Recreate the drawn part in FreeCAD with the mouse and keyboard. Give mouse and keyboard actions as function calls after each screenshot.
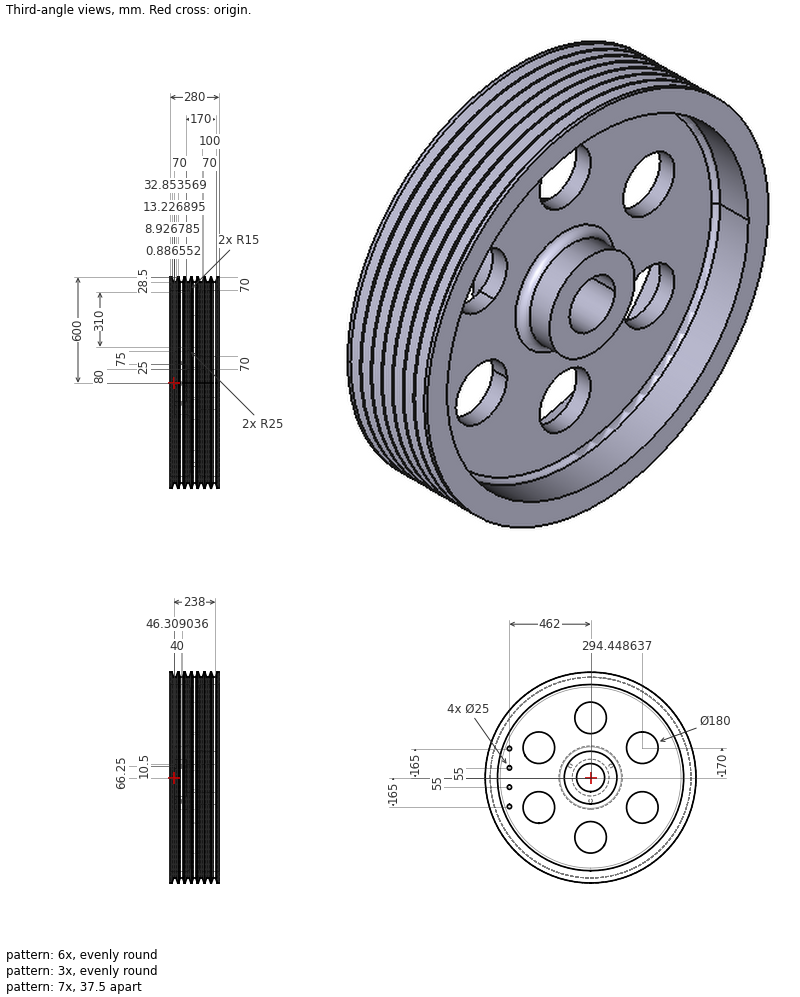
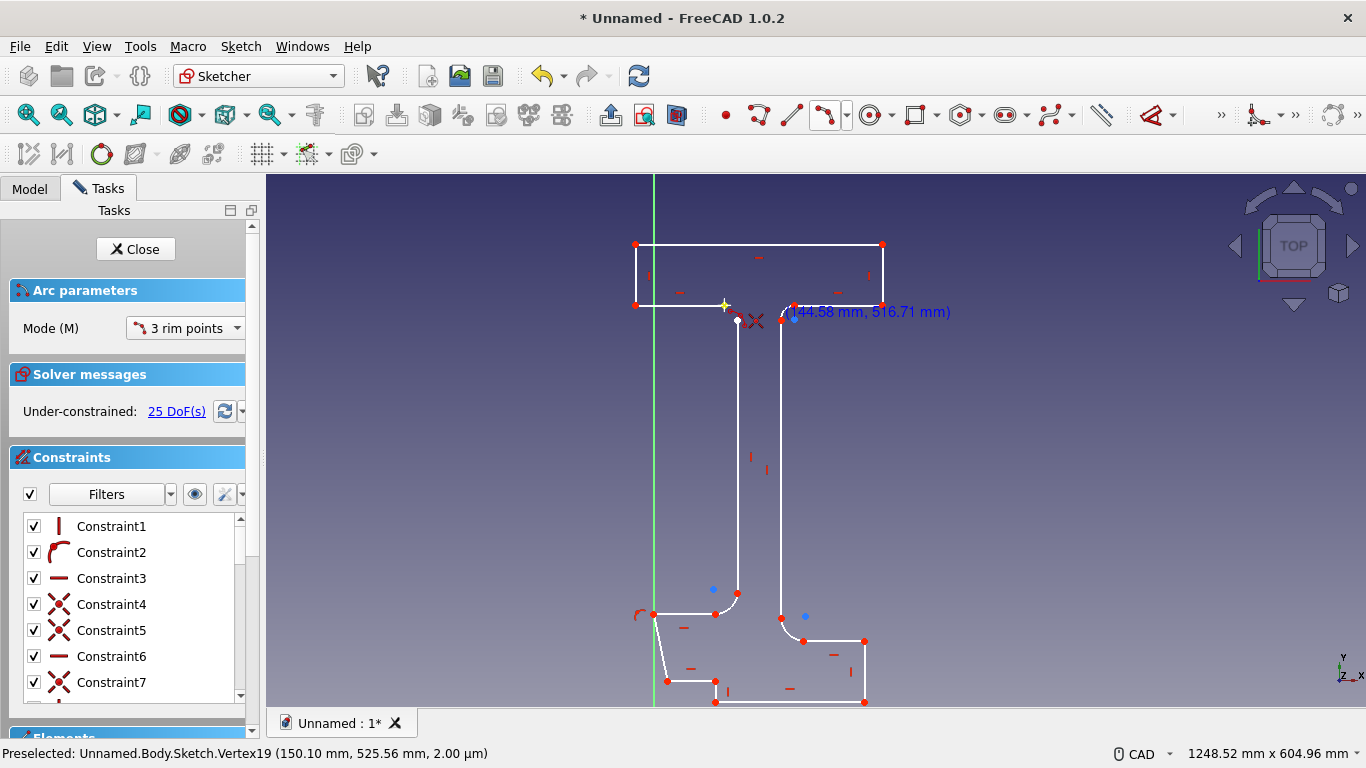
click(725, 306)
click(738, 320)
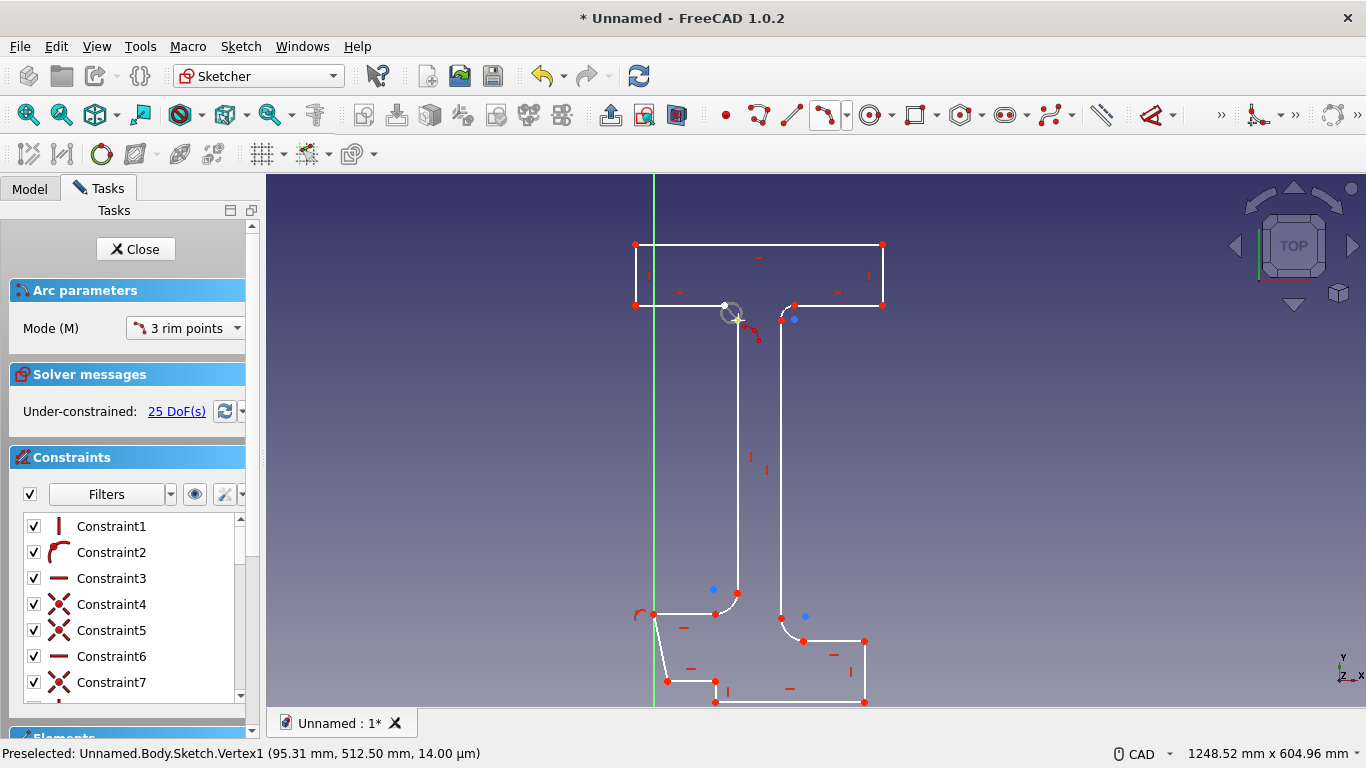
scroll(734, 309, up, 8)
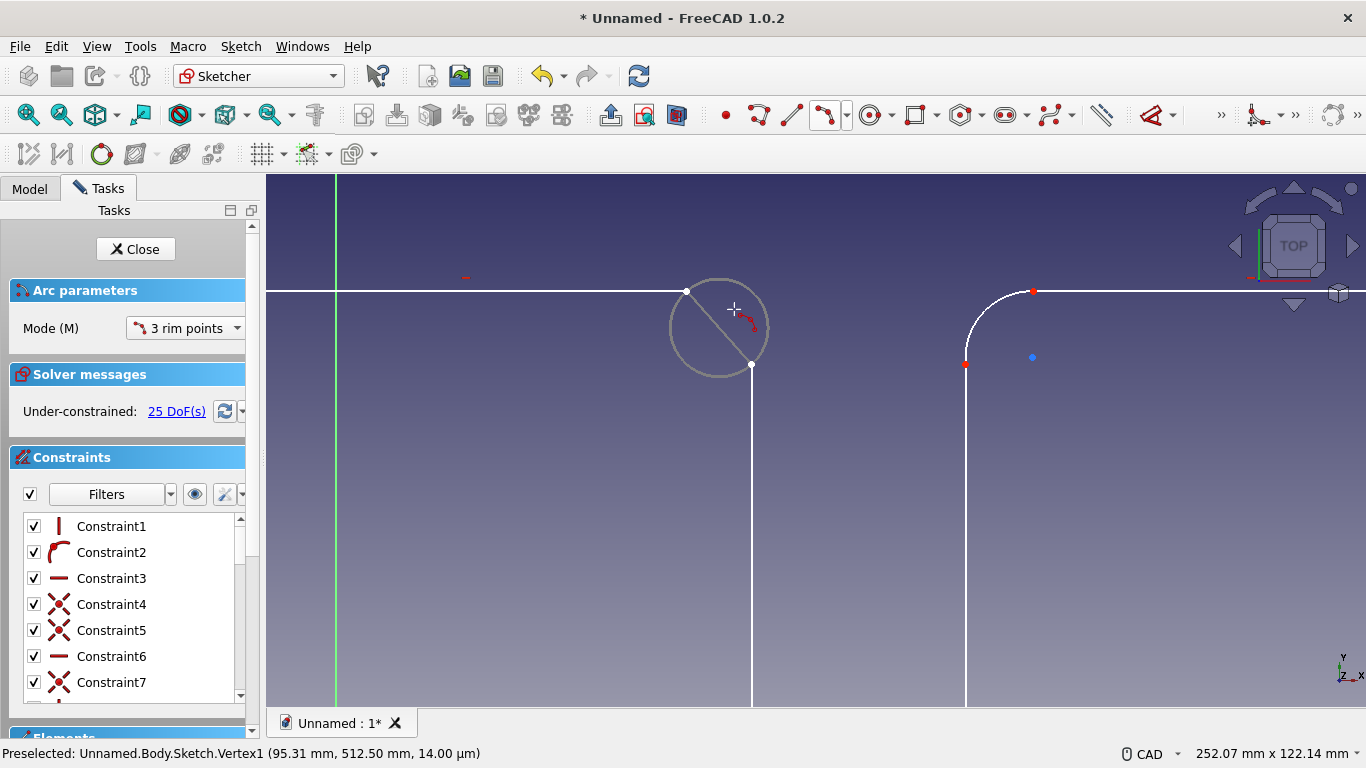
click(731, 307)
key(Escape)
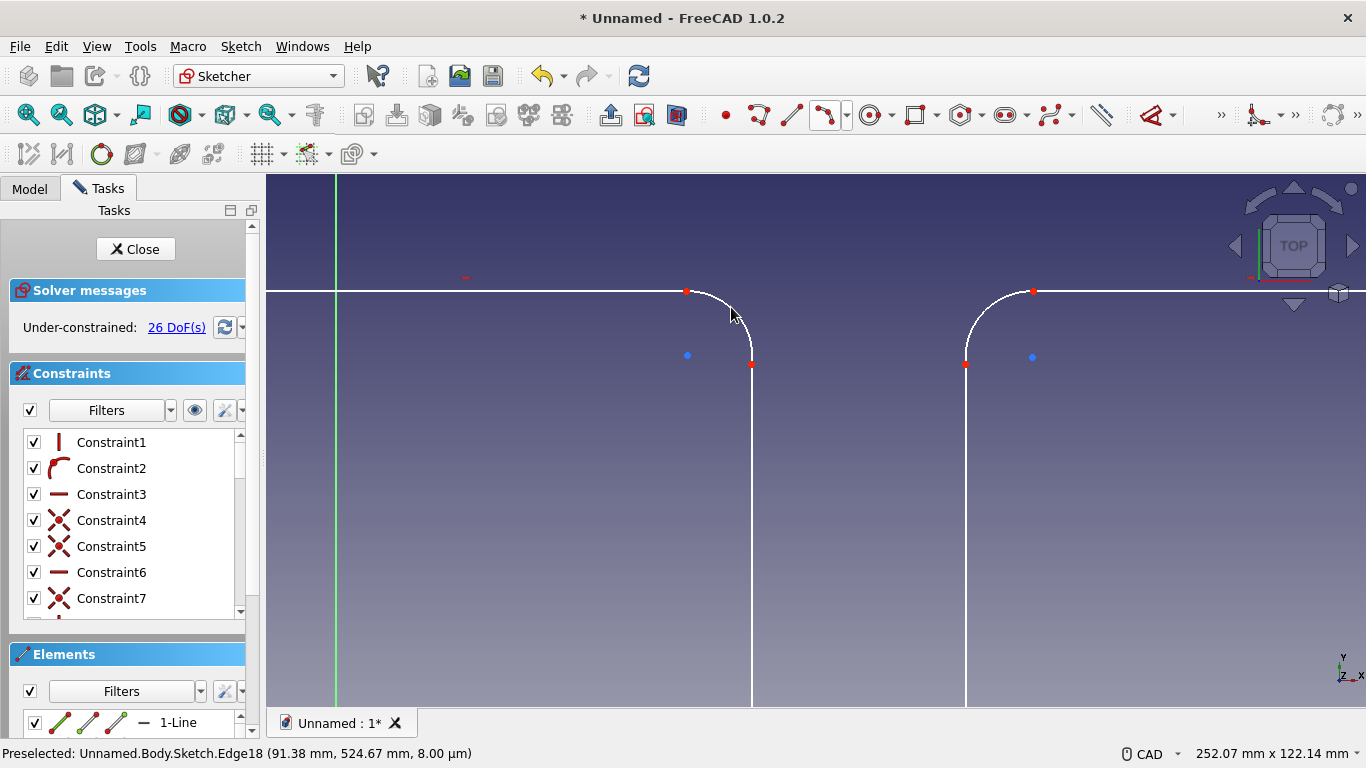
scroll(730, 307, down, 10)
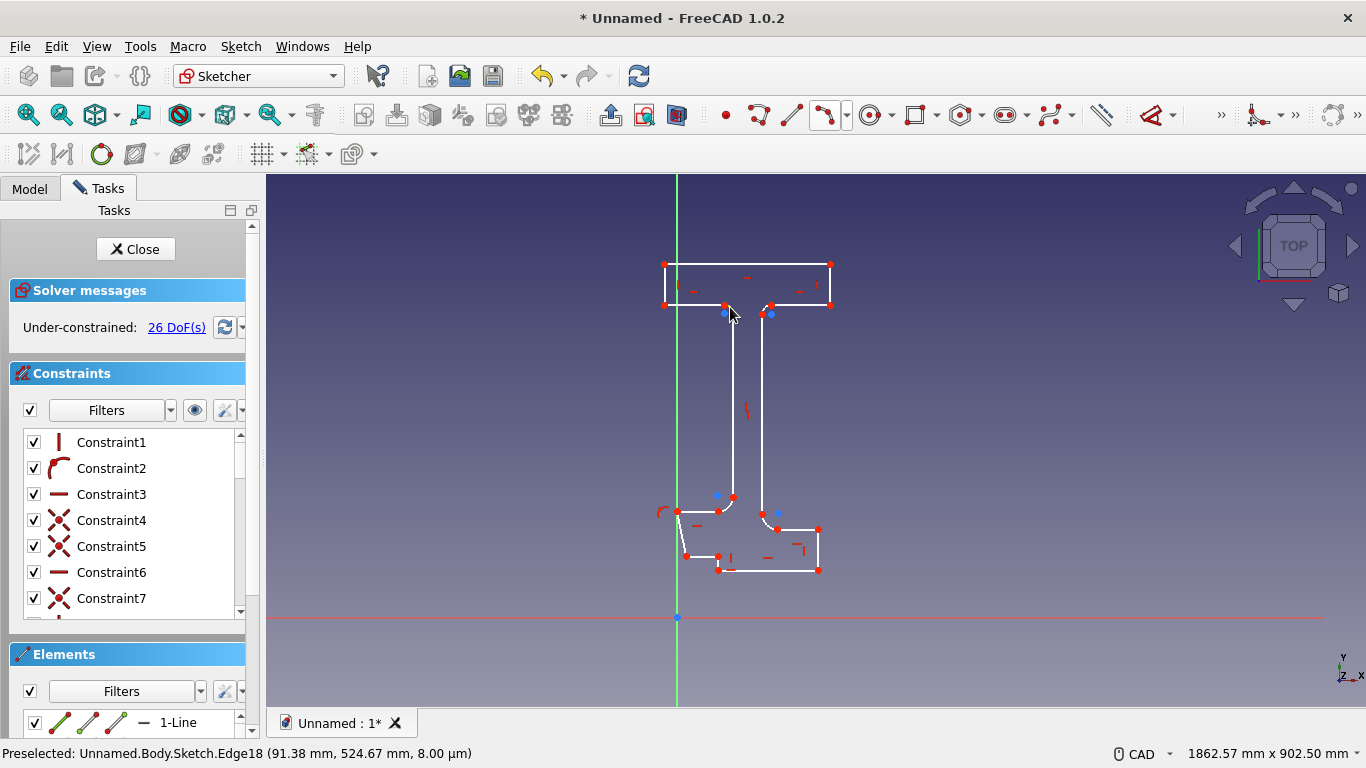
click(733, 352)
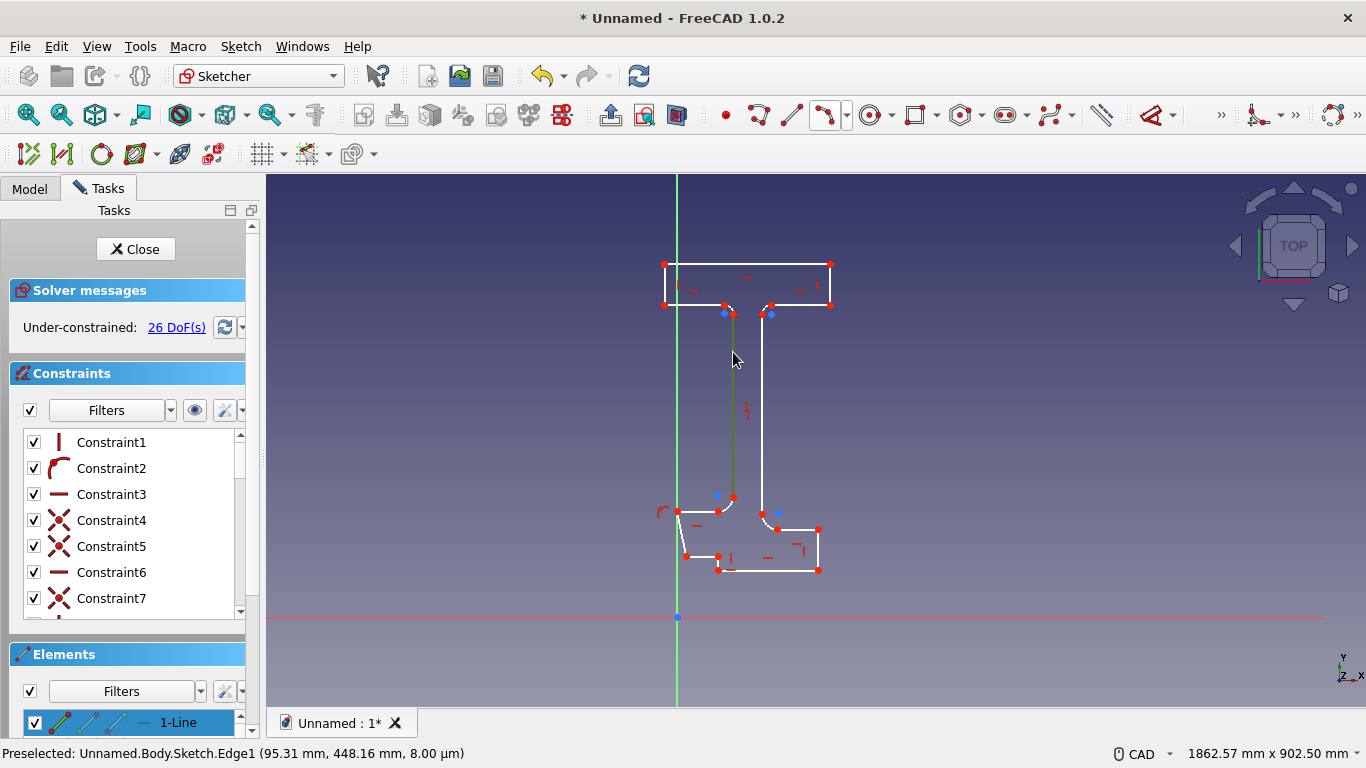
scroll(728, 508, up, 2)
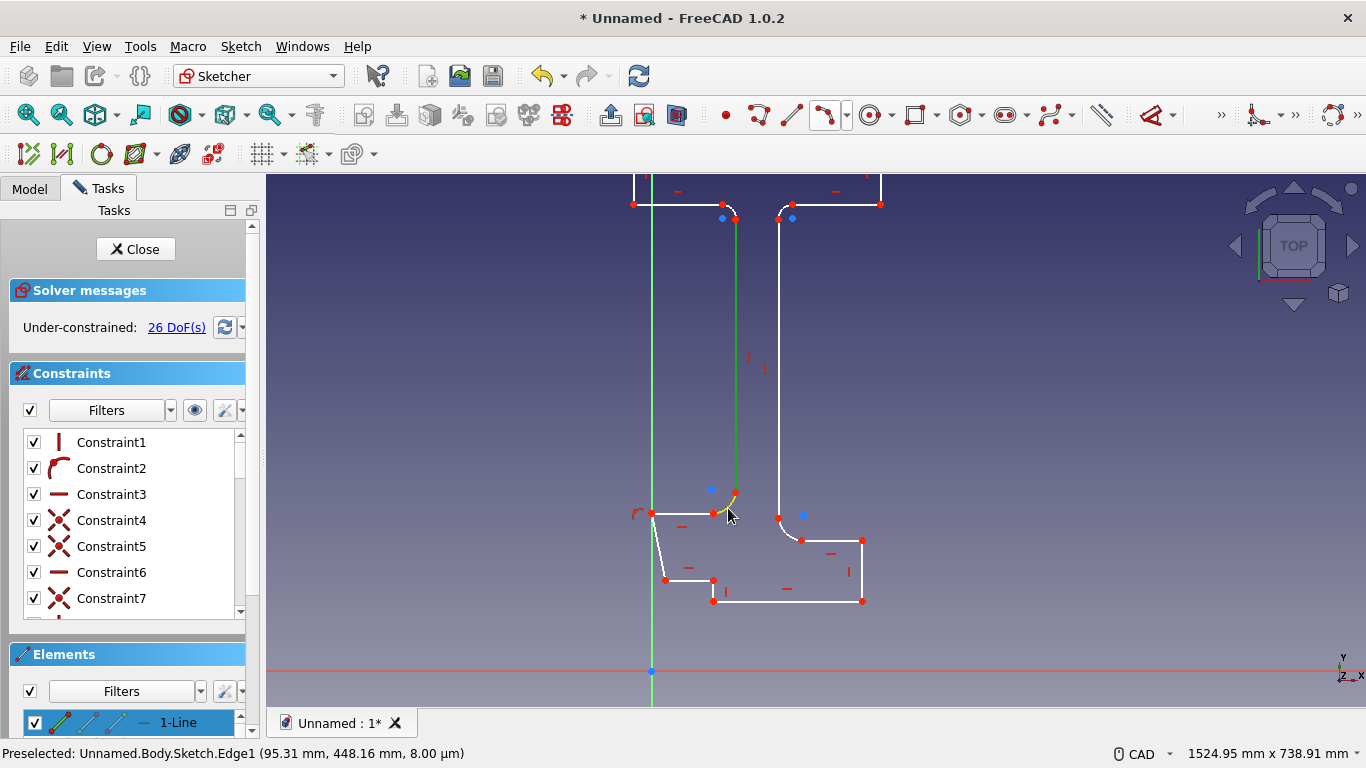
click(728, 507)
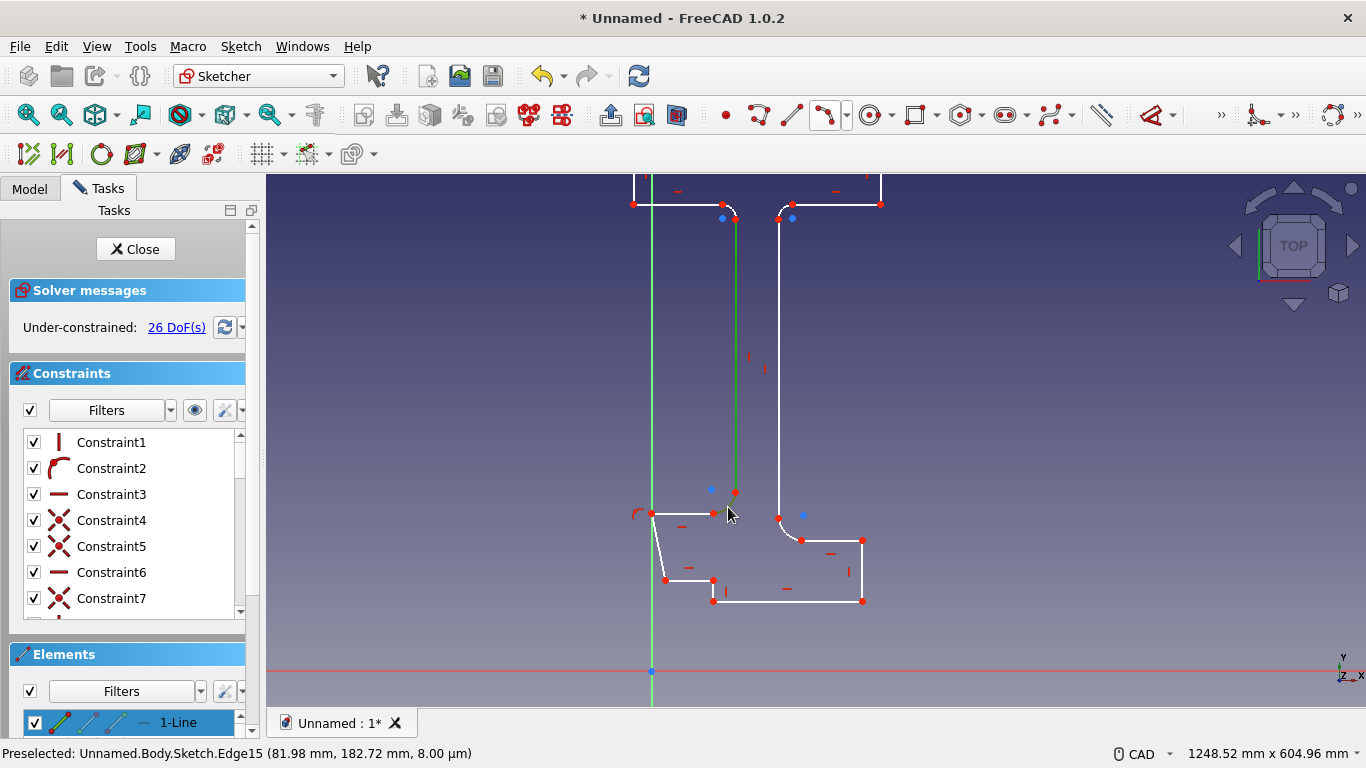
key(t)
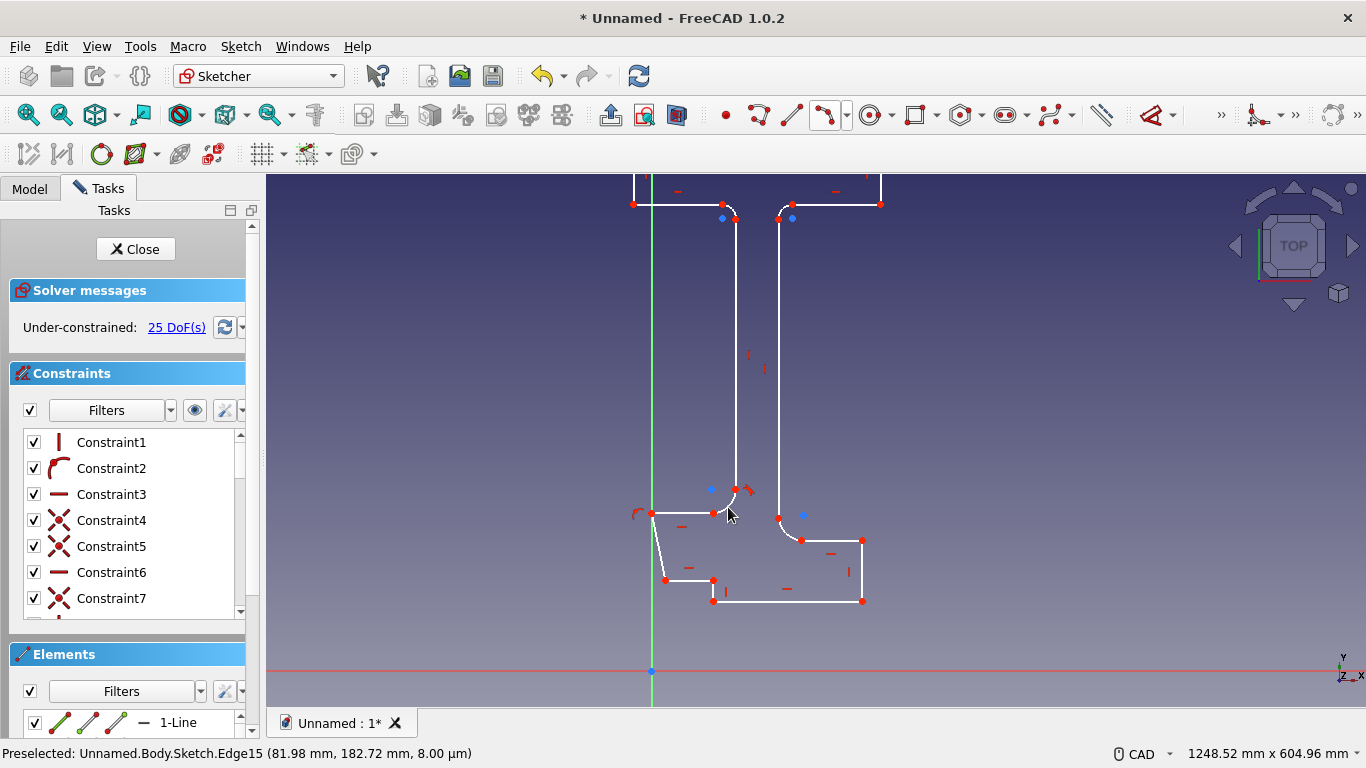
click(736, 301)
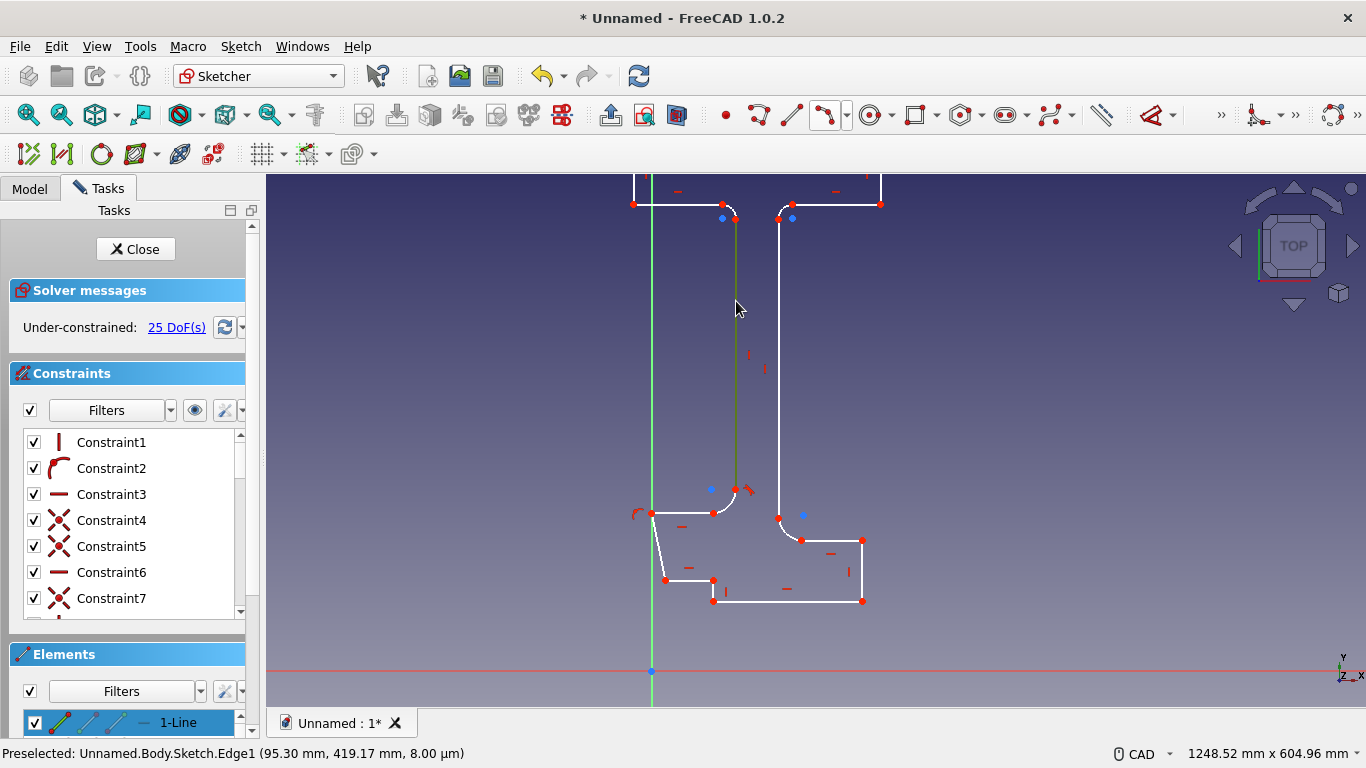
scroll(733, 209, up, 2)